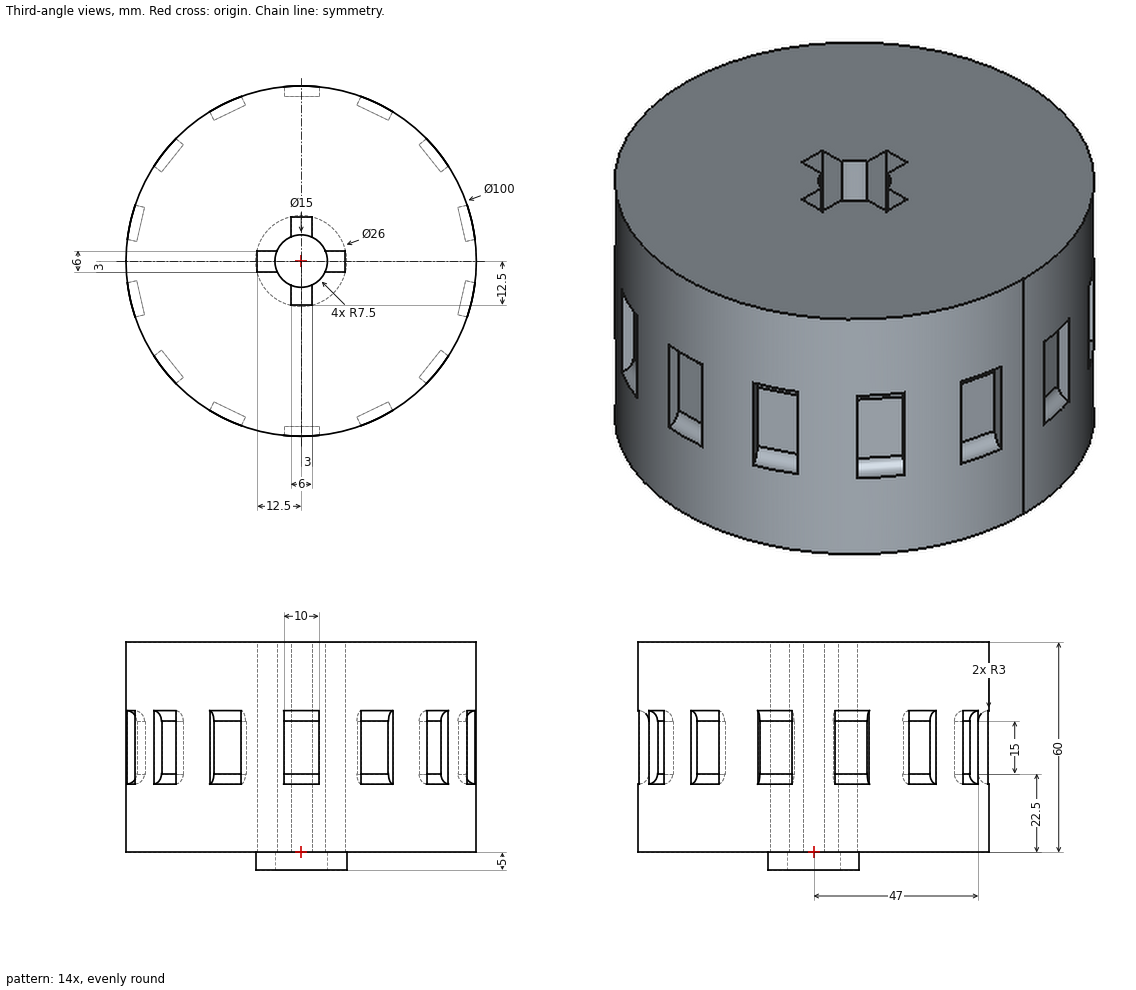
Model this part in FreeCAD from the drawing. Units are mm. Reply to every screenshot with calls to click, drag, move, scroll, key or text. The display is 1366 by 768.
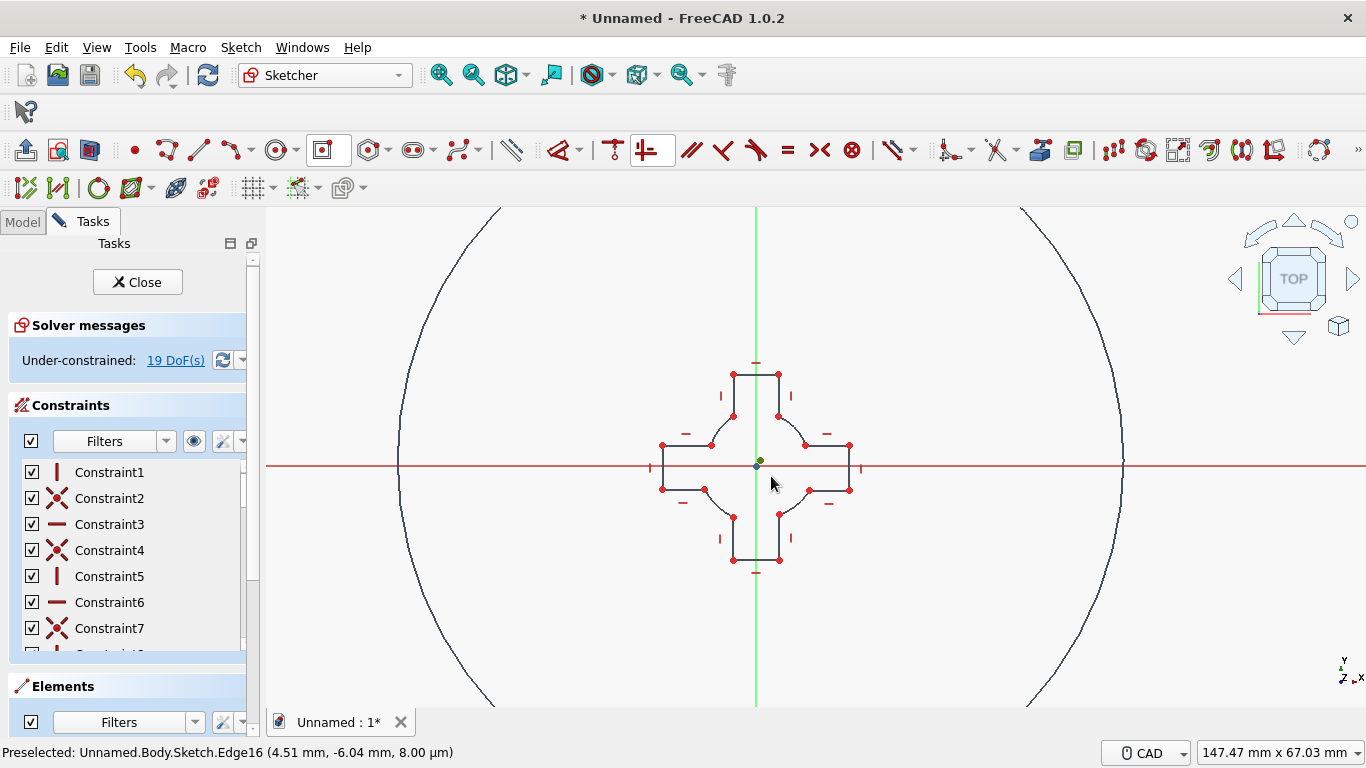
click(614, 150)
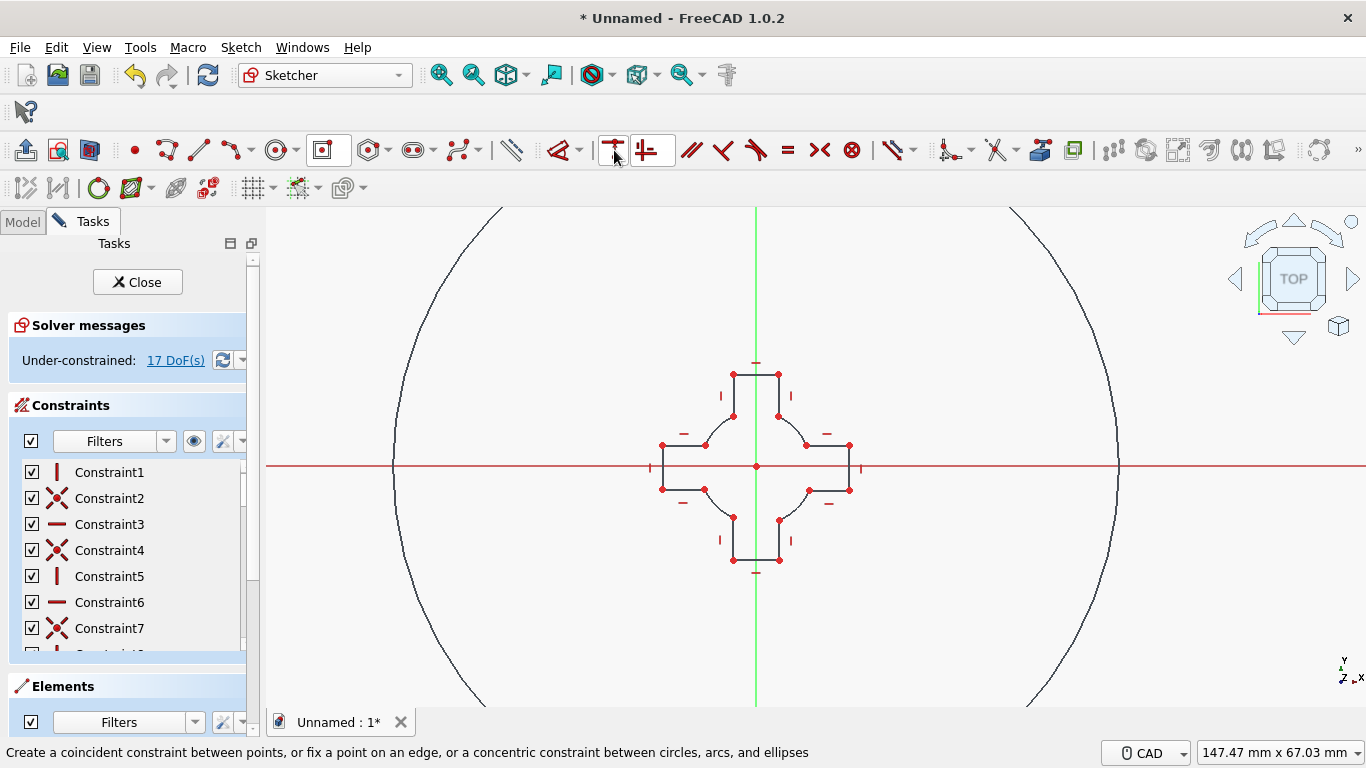
click(711, 500)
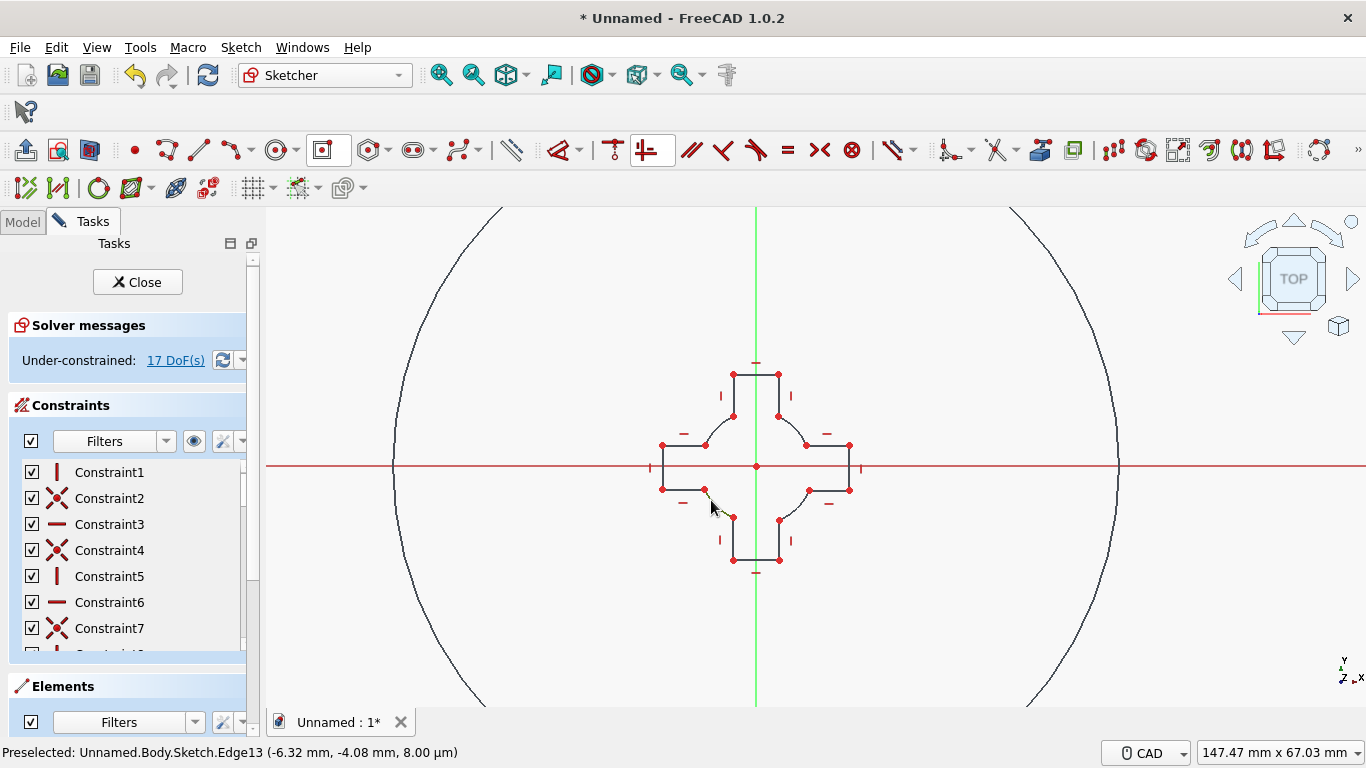
click(723, 423)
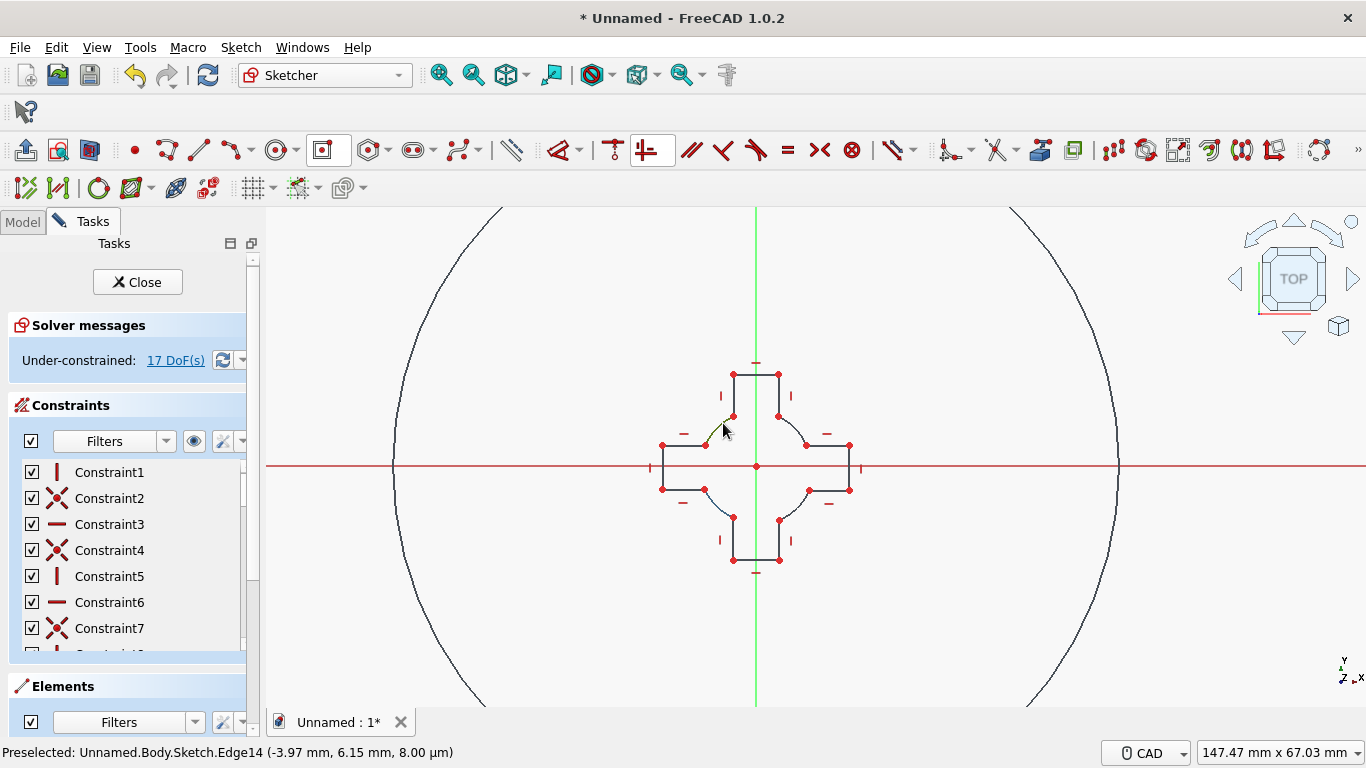
click(800, 435)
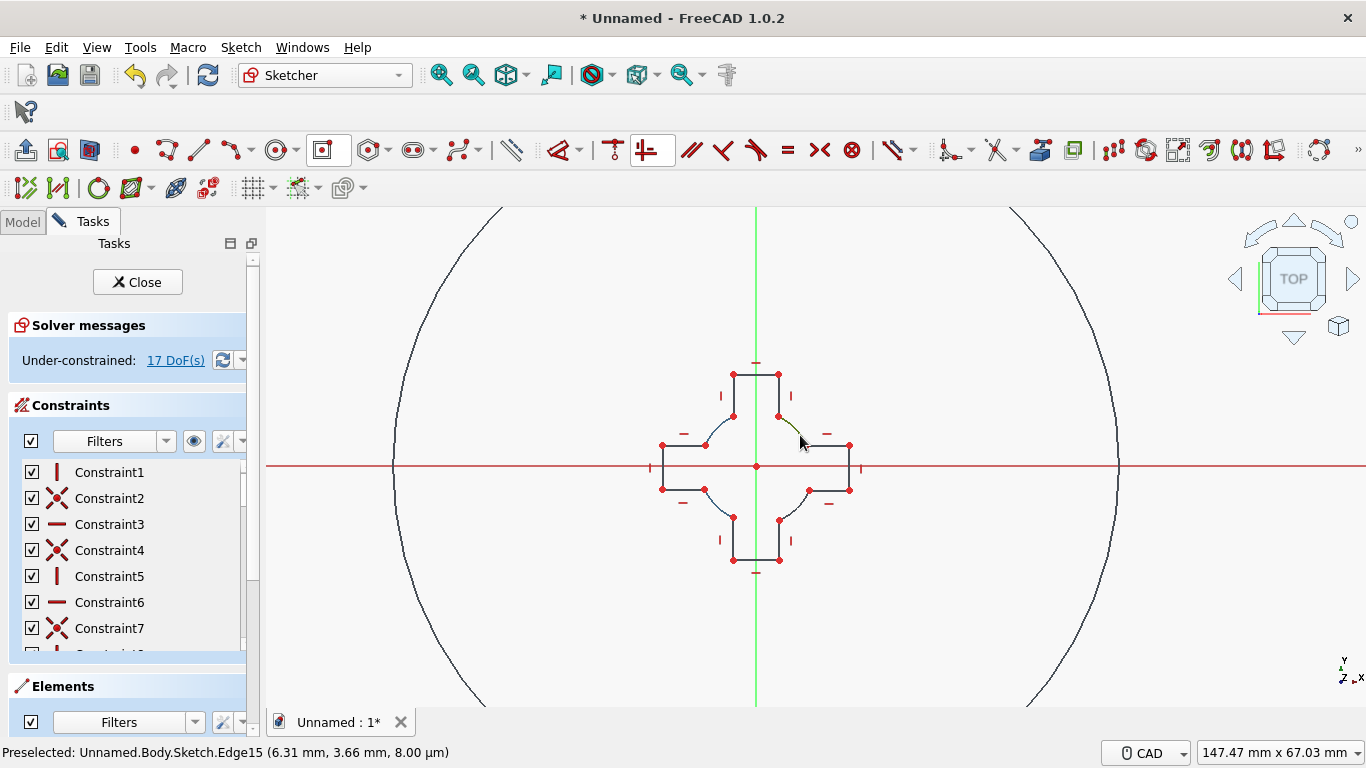
click(790, 514)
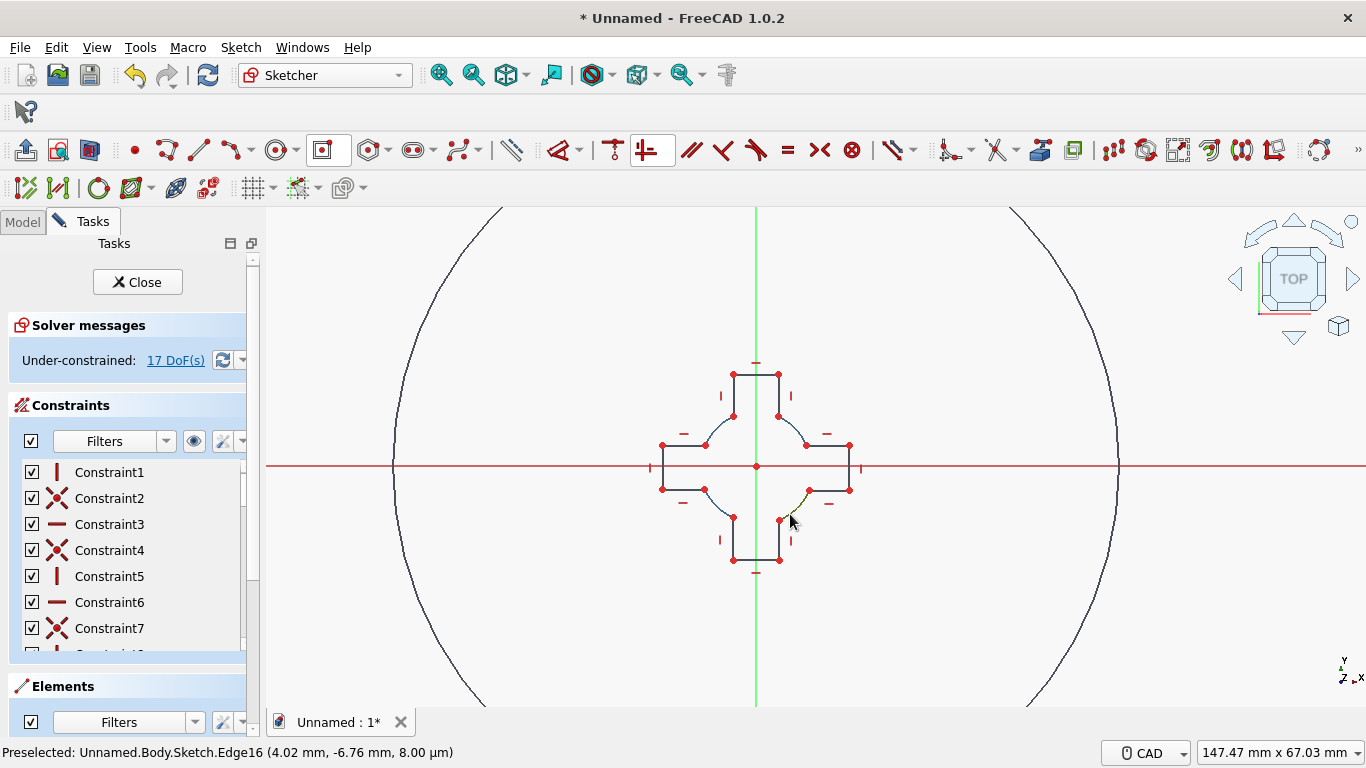
click(788, 150)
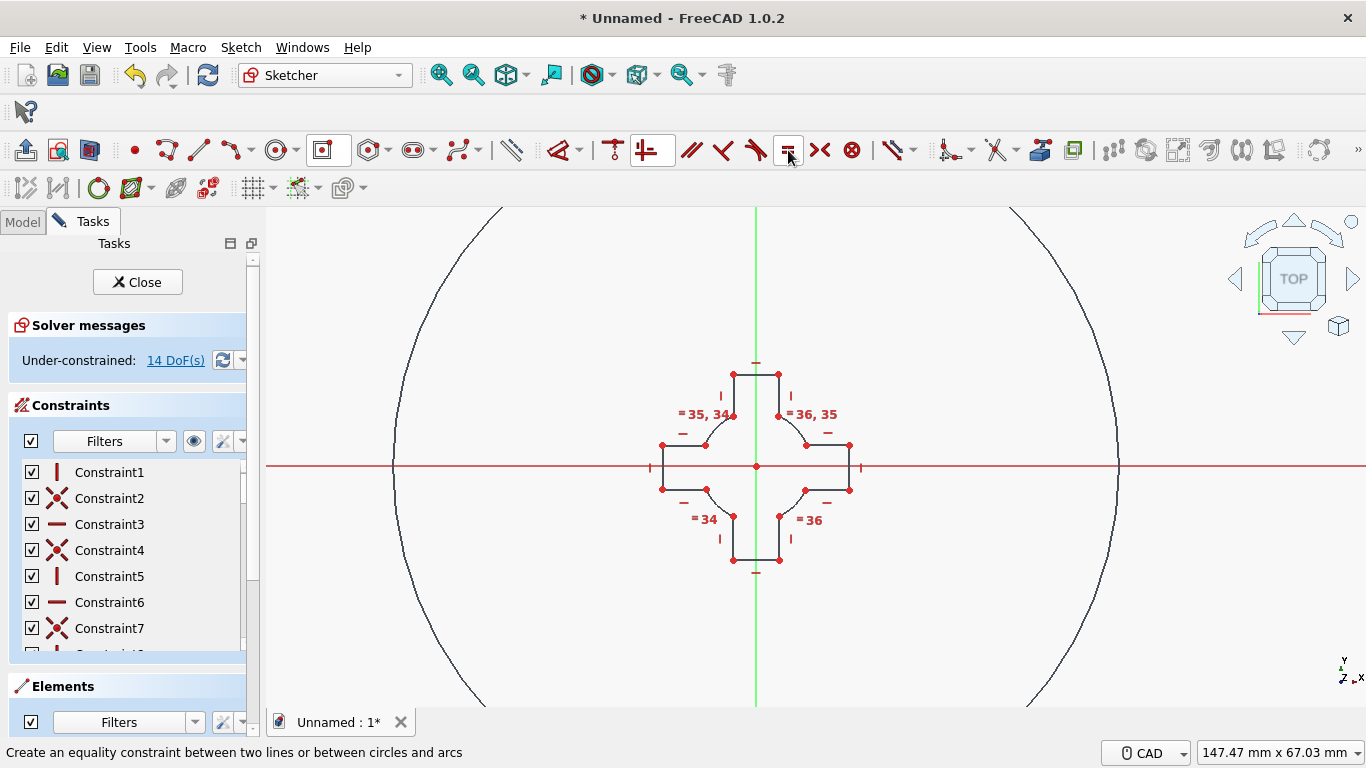
click(733, 560)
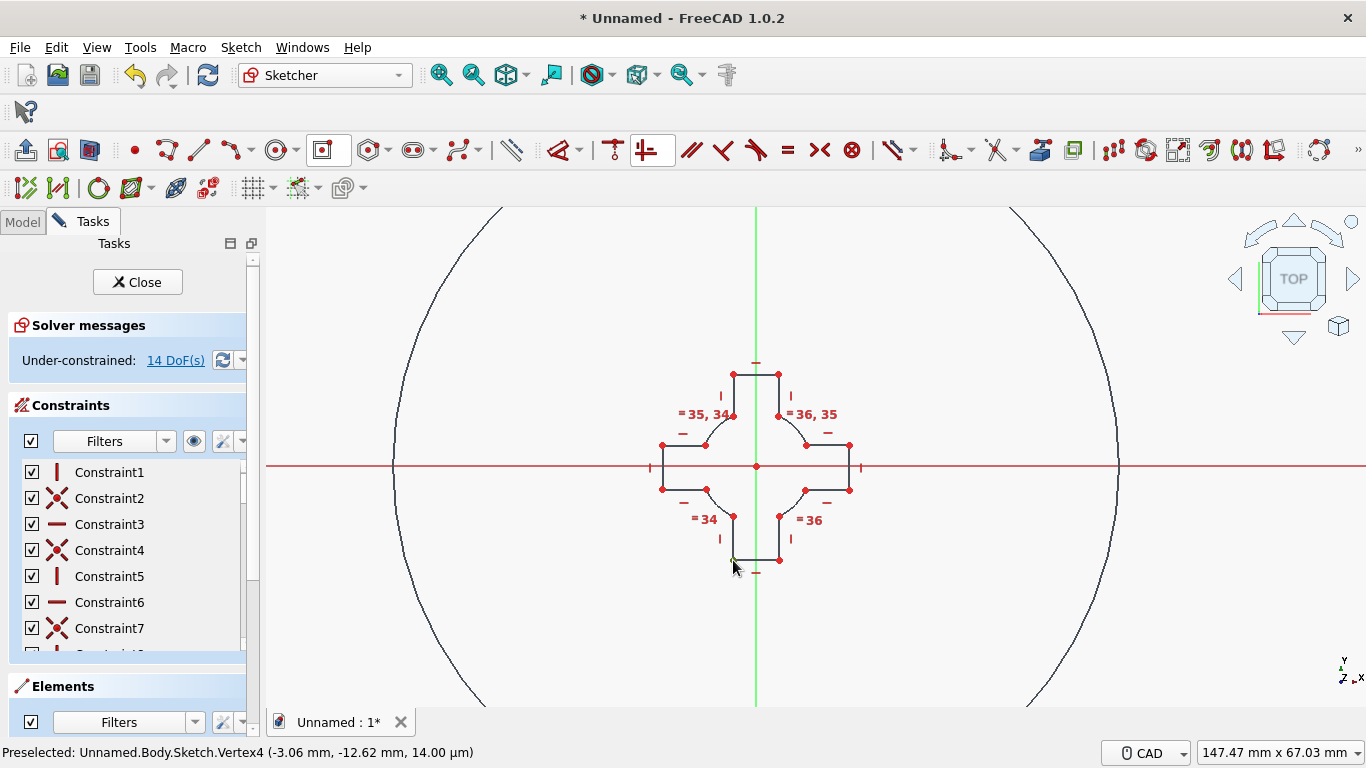
click(734, 375)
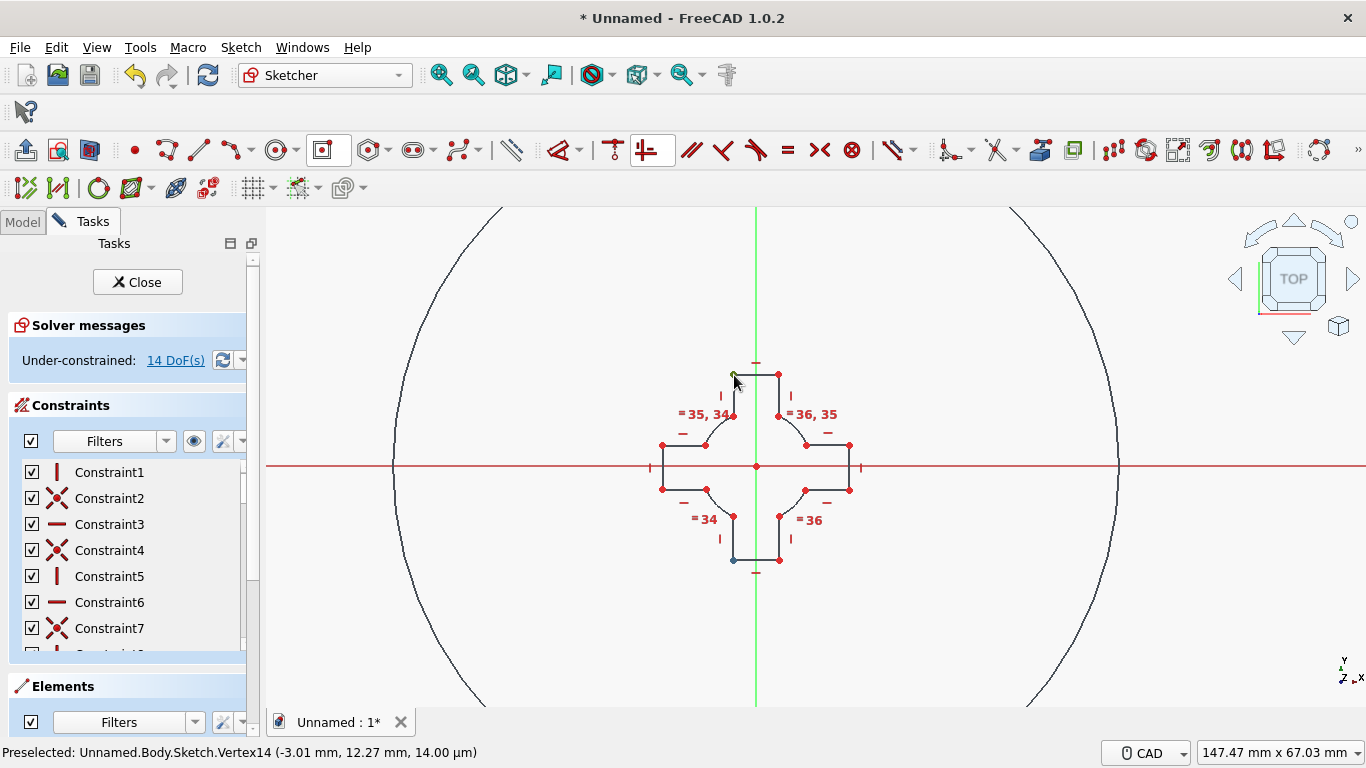
click(359, 466)